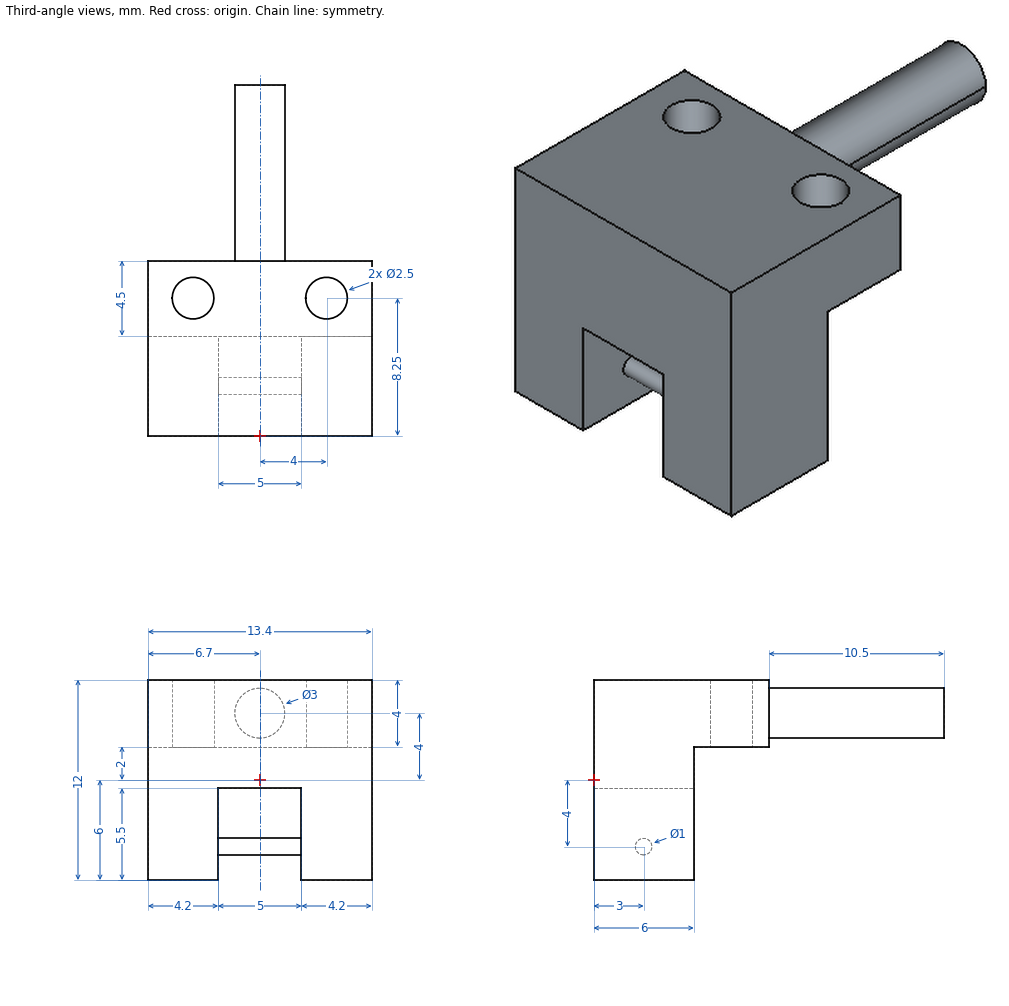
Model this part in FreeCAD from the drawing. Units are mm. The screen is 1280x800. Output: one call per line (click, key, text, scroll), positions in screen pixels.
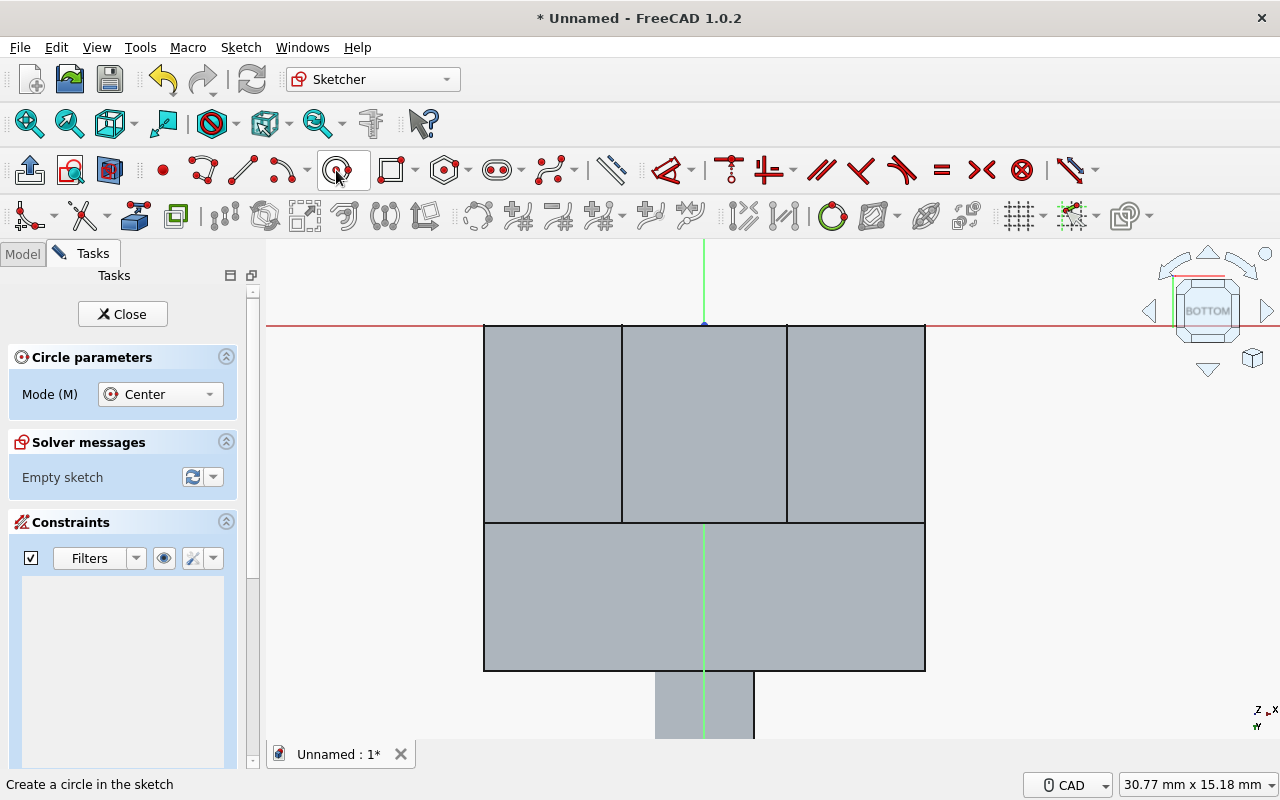
click(836, 597)
move(865, 568)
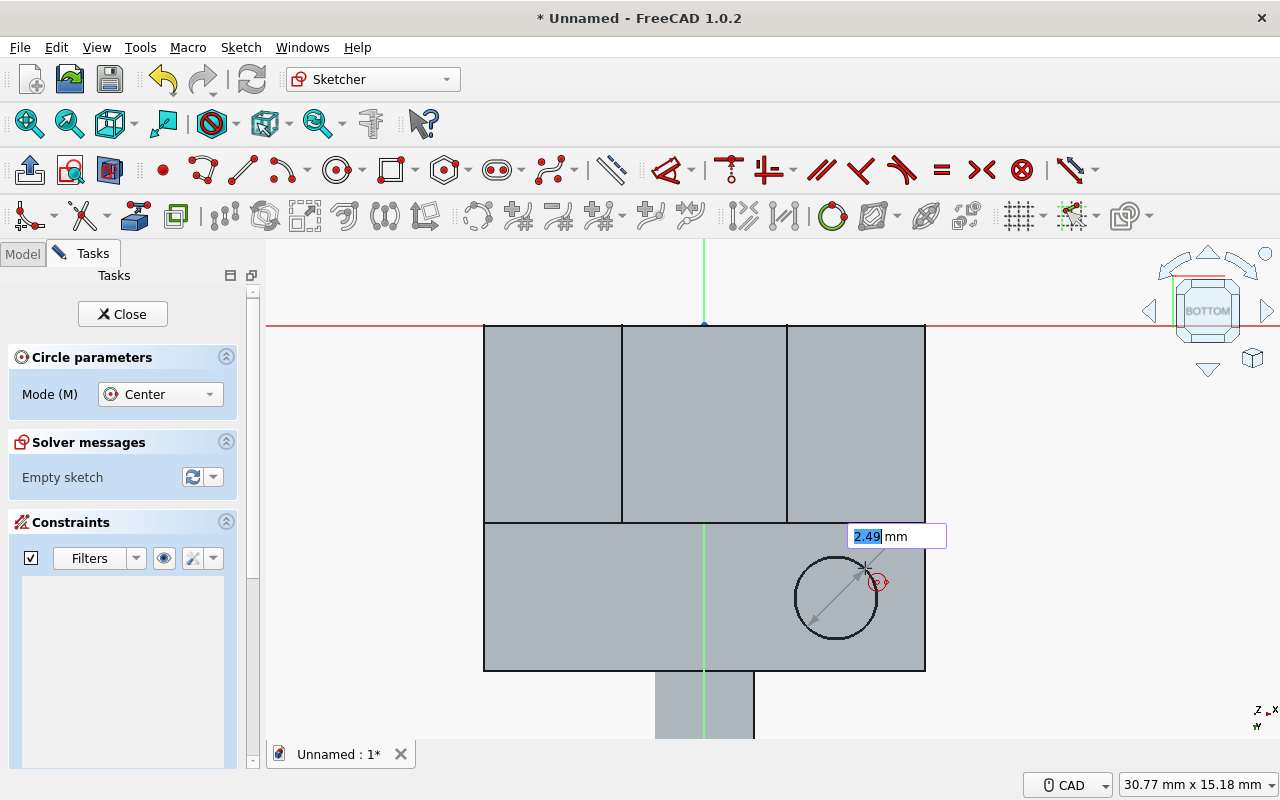
text(2.5)
key(Return)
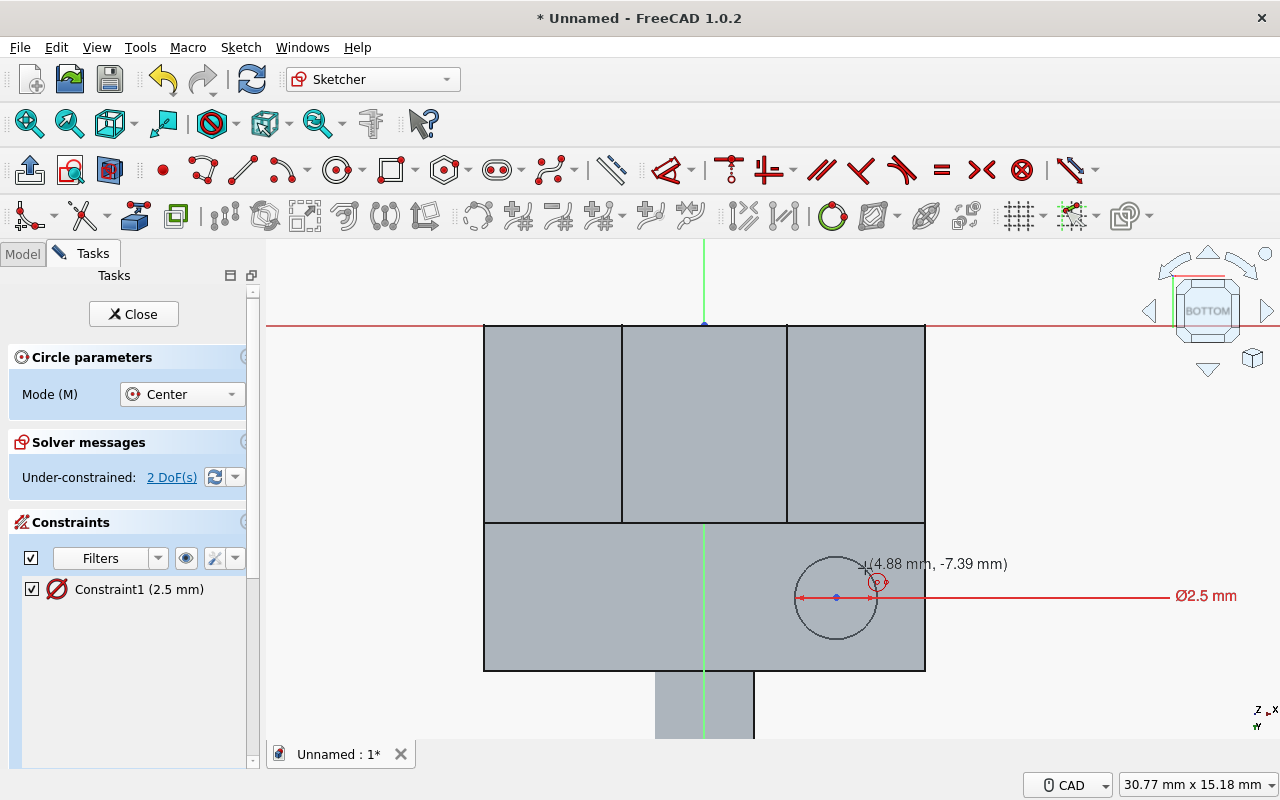
click(572, 597)
move(602, 568)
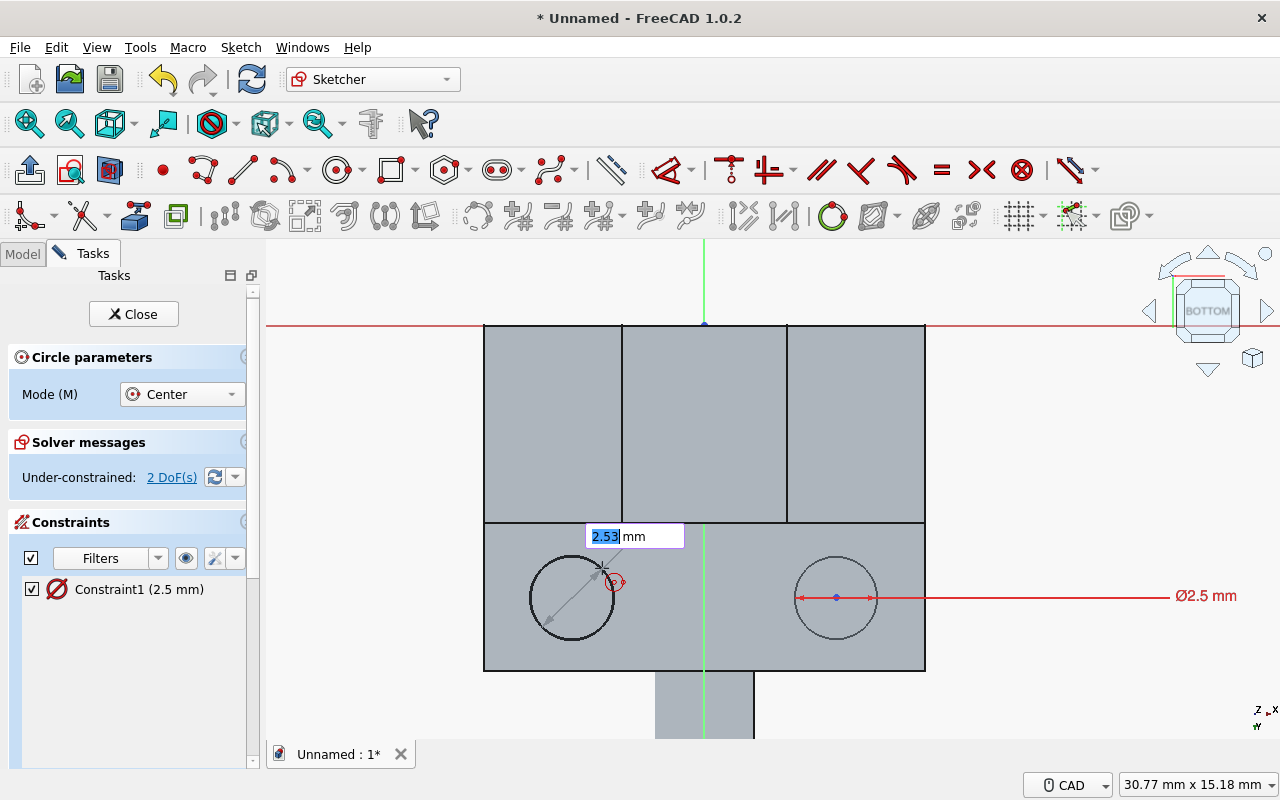
text(2.5)
key(Return)
key(Escape)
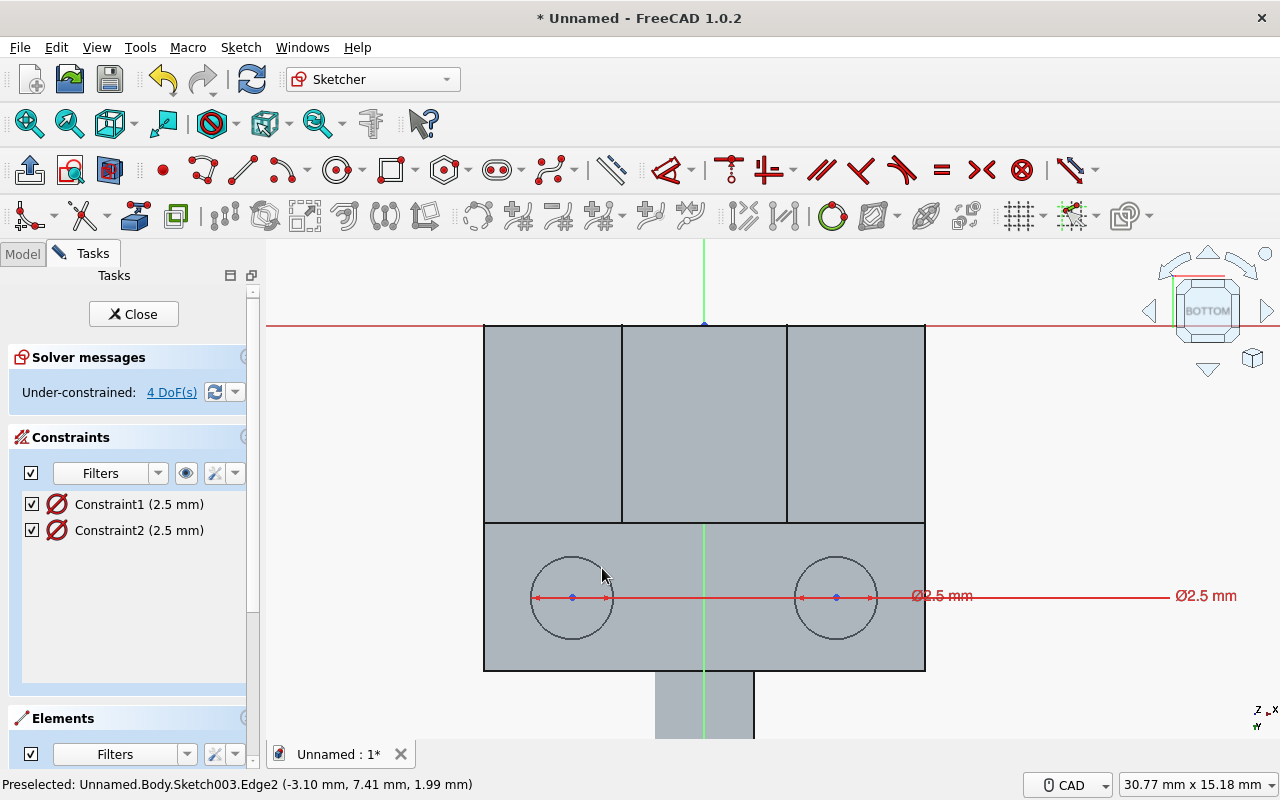
click(836, 598)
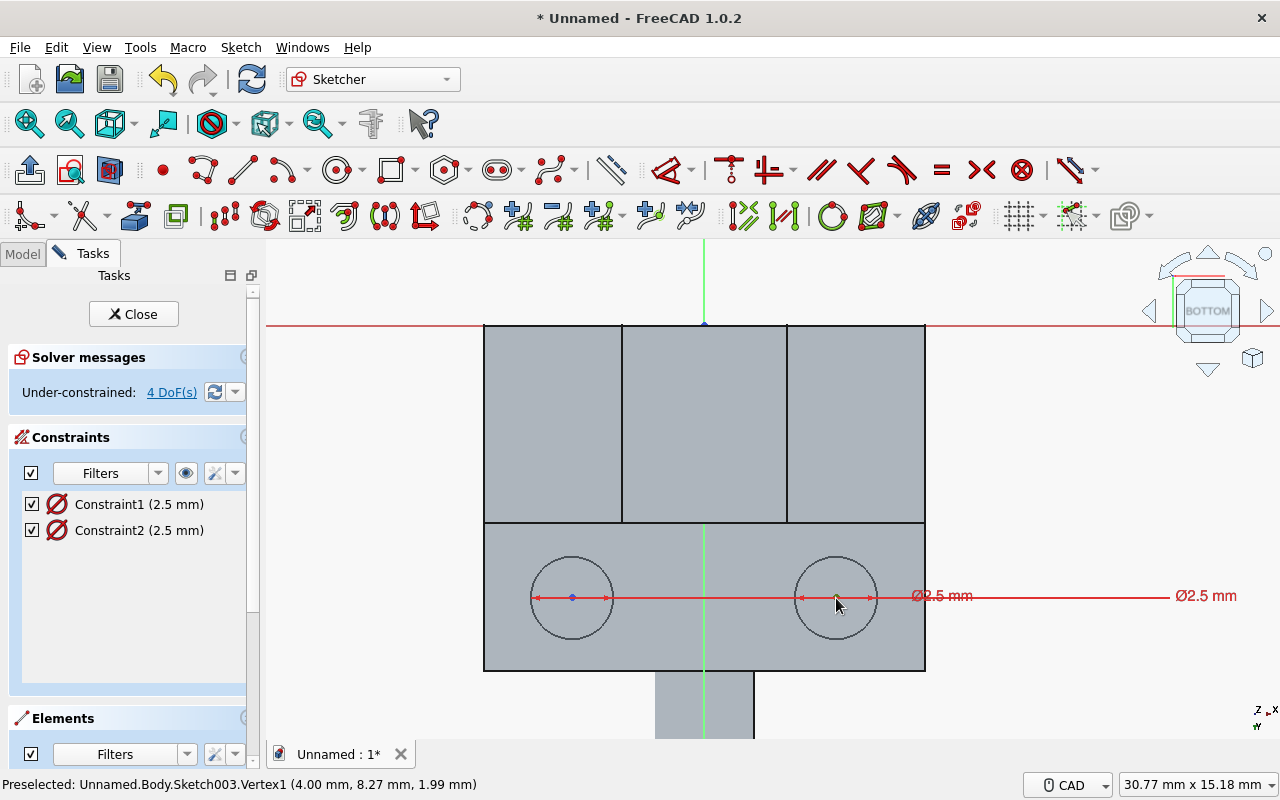
click(572, 598)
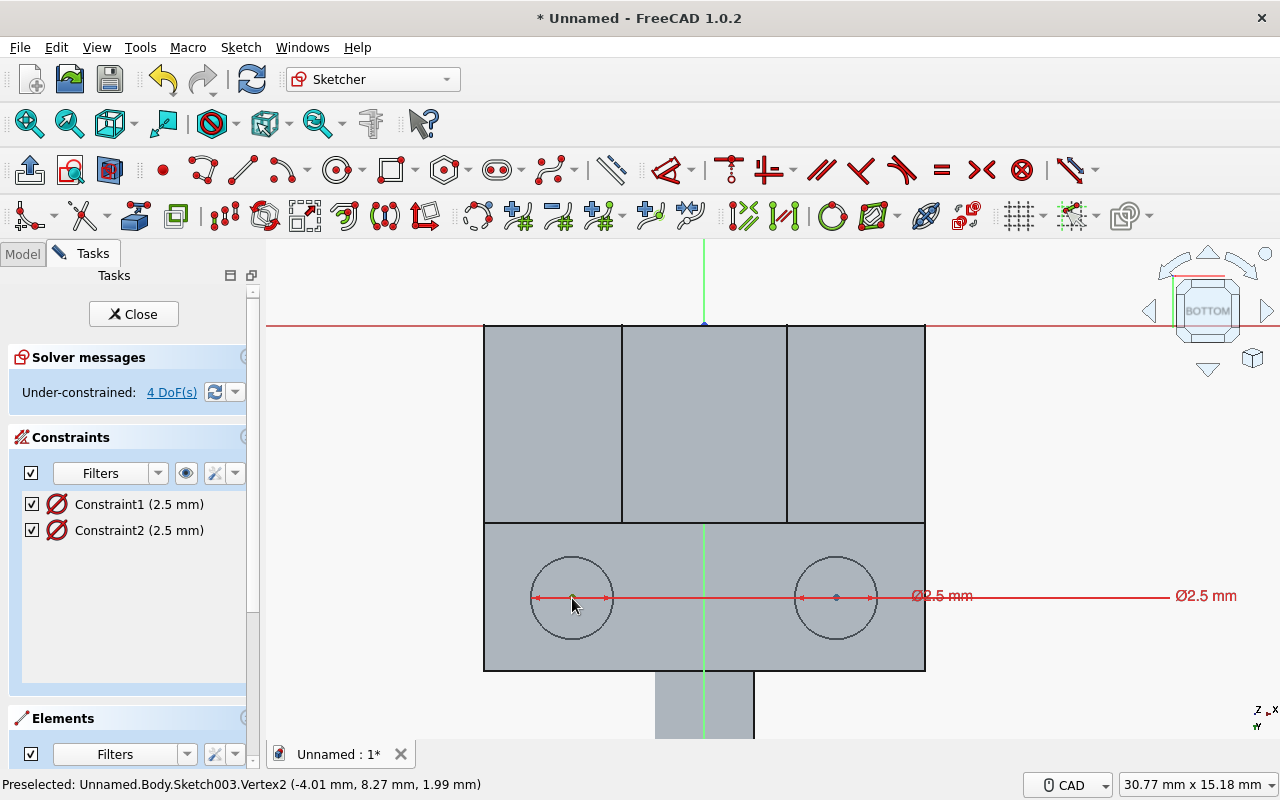
click(704, 679)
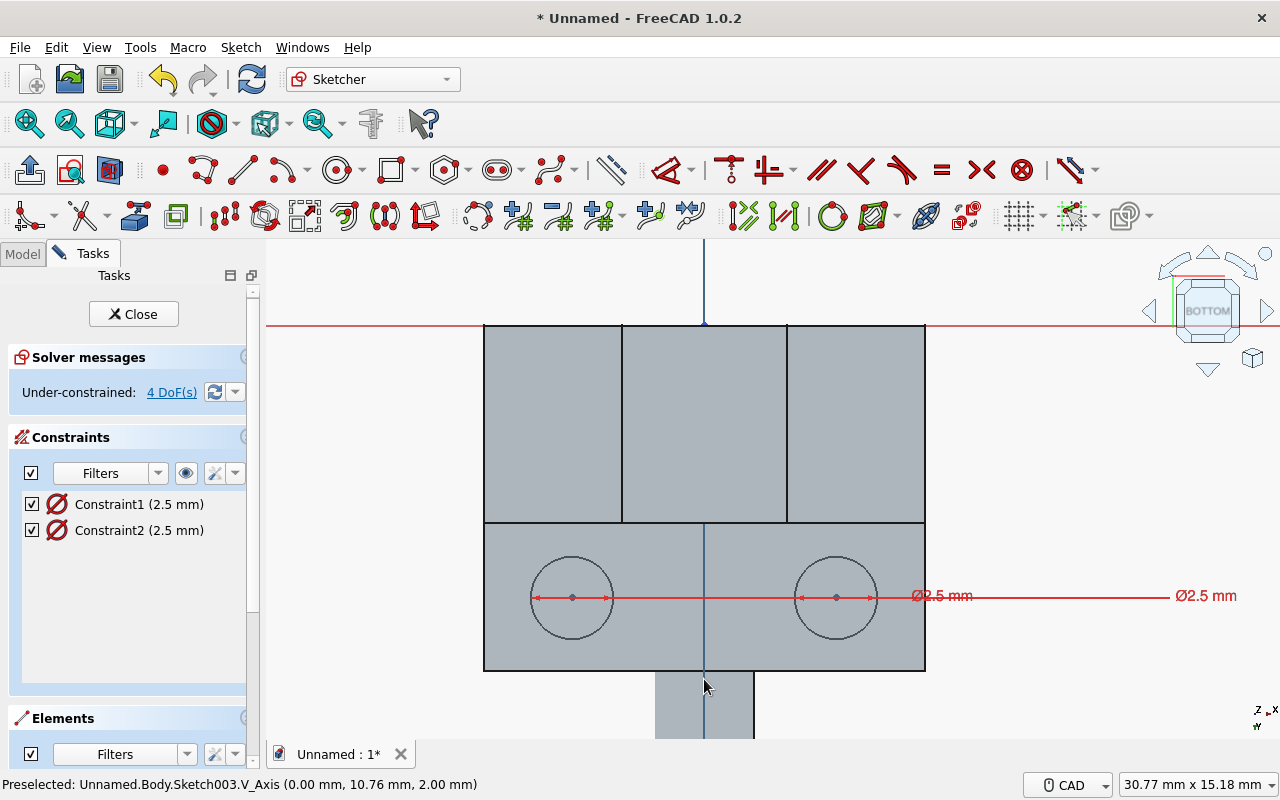
click(982, 170)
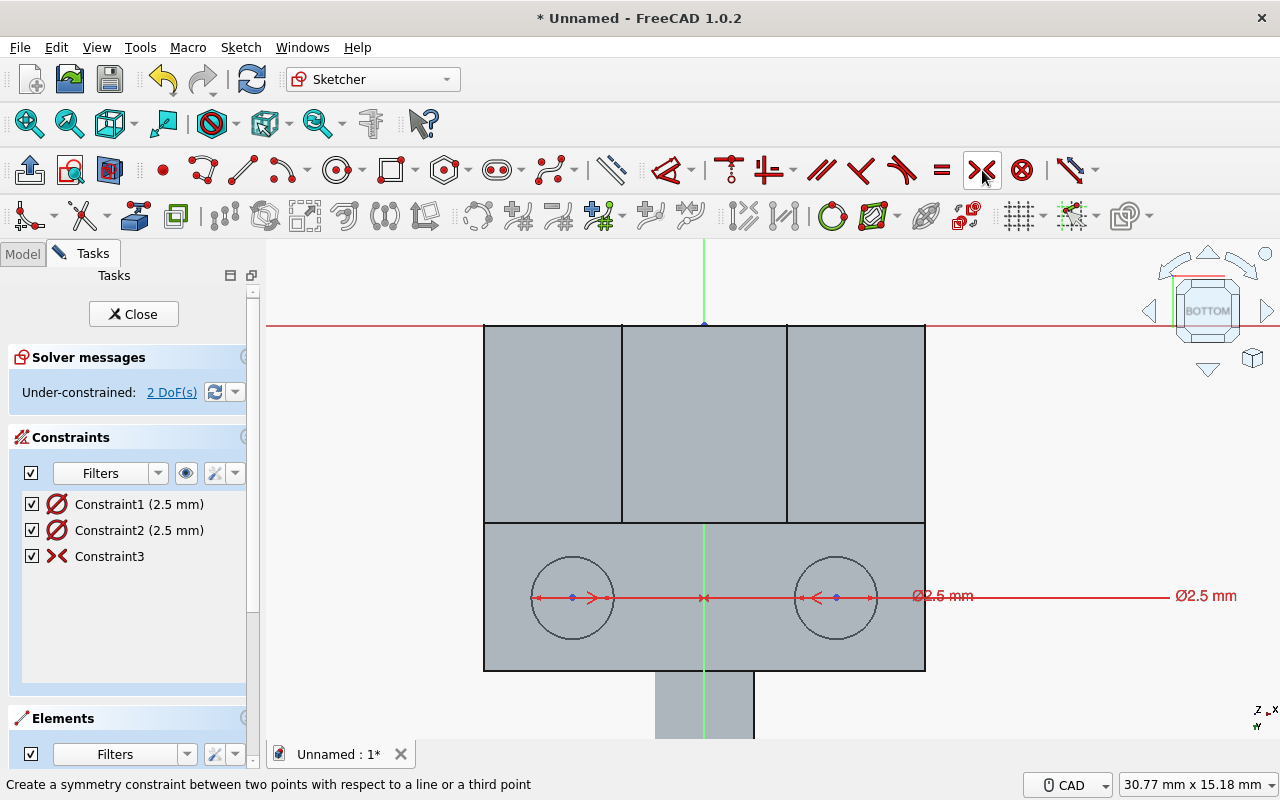
click(666, 170)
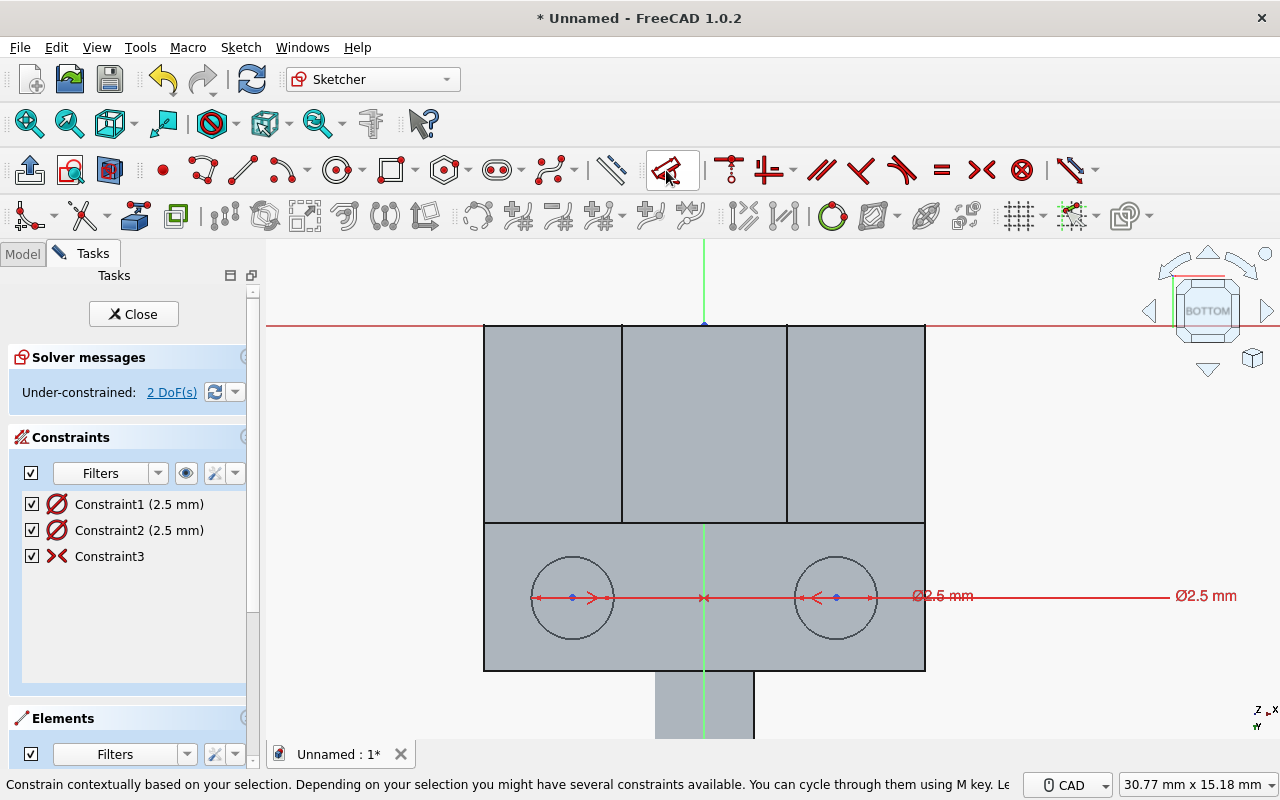
click(836, 598)
click(770, 292)